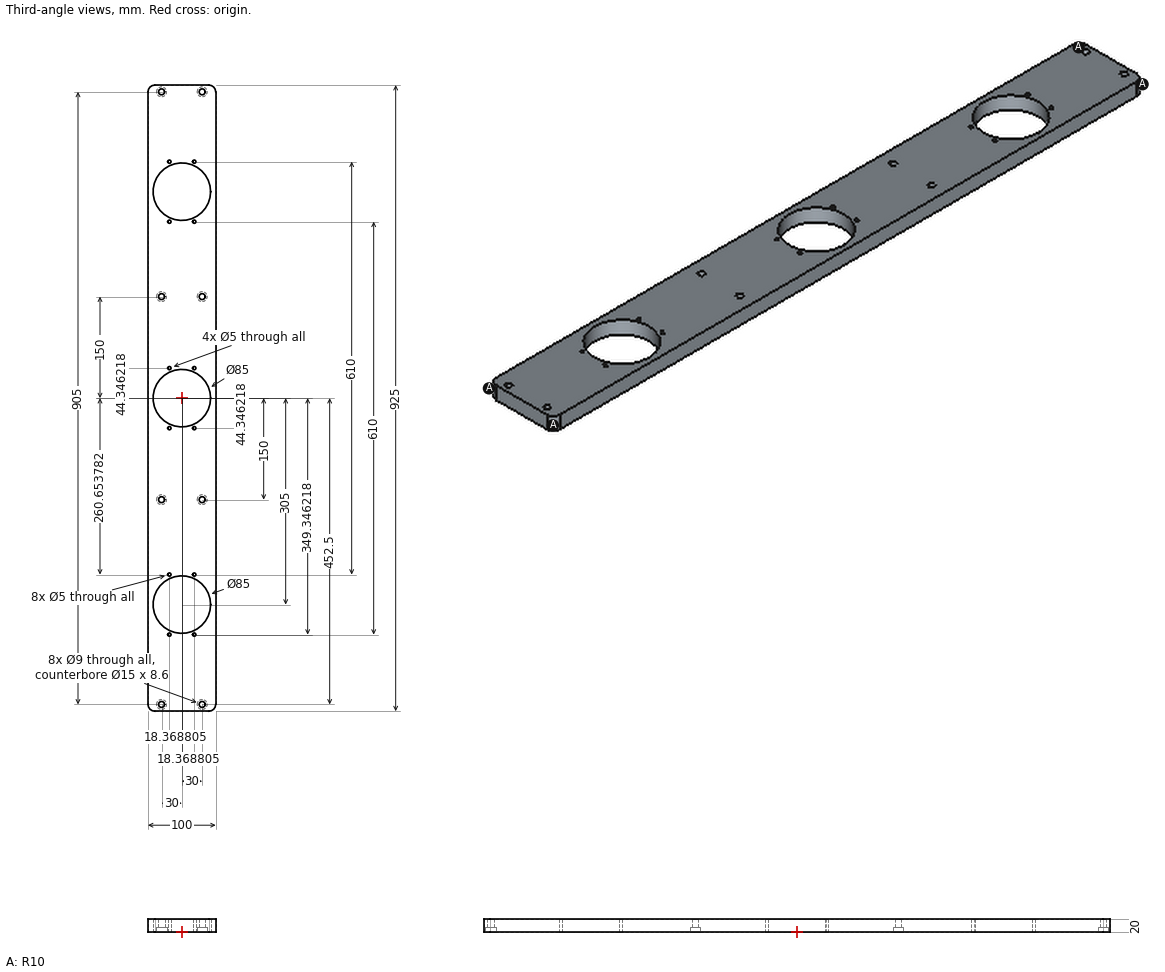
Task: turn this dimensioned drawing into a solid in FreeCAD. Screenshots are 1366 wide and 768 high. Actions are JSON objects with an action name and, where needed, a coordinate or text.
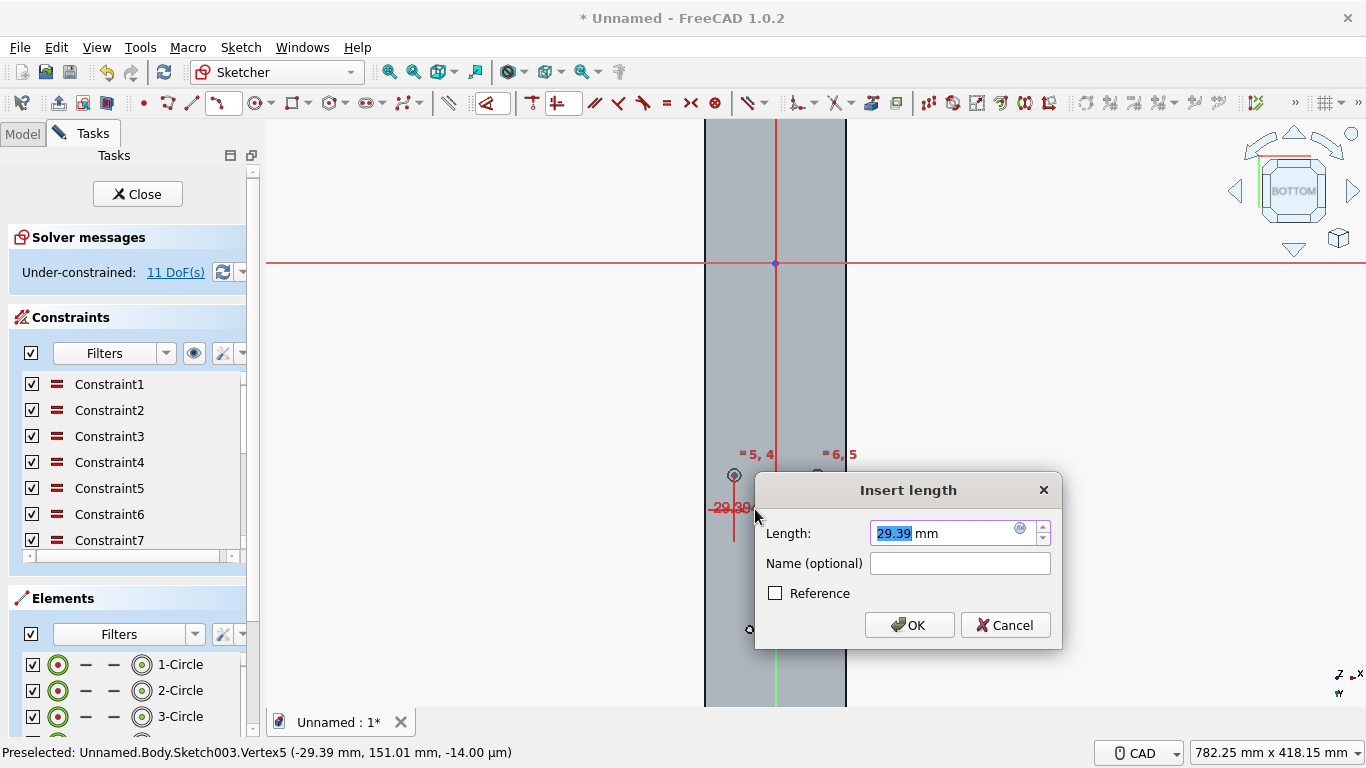
{"action": "type", "text": "30"}
{"action": "key", "text": "Return"}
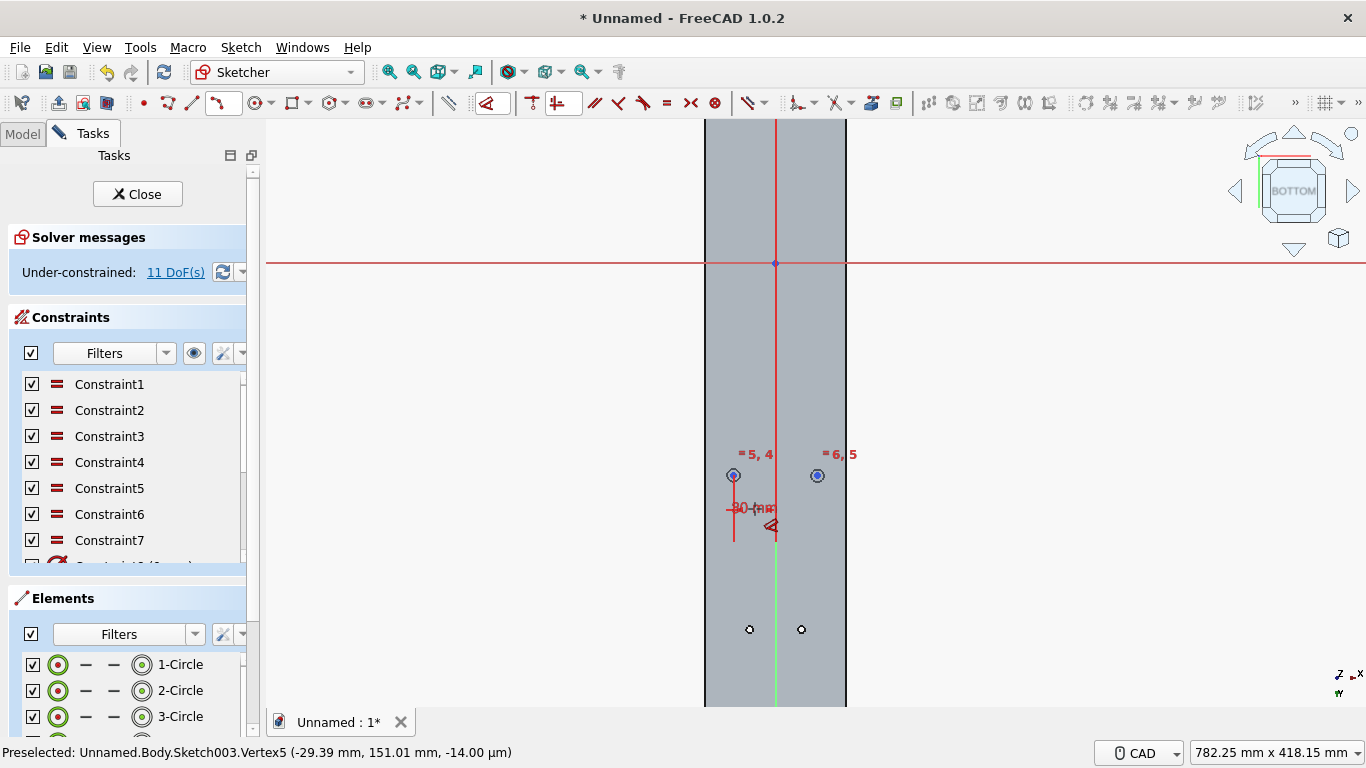
{"action": "left_click", "coordinate": [818, 476]}
{"action": "left_click", "coordinate": [797, 229]}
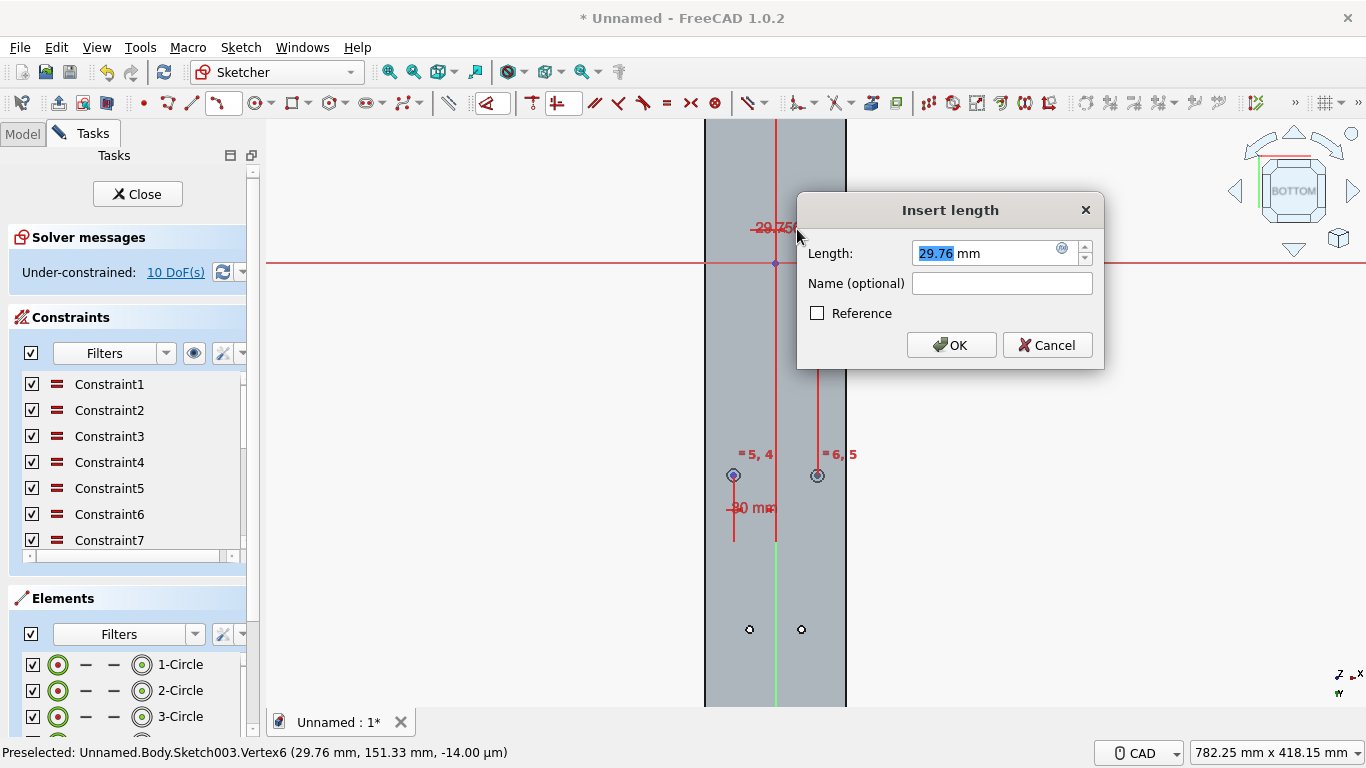
{"action": "type", "text": "30"}
{"action": "key", "text": "Return"}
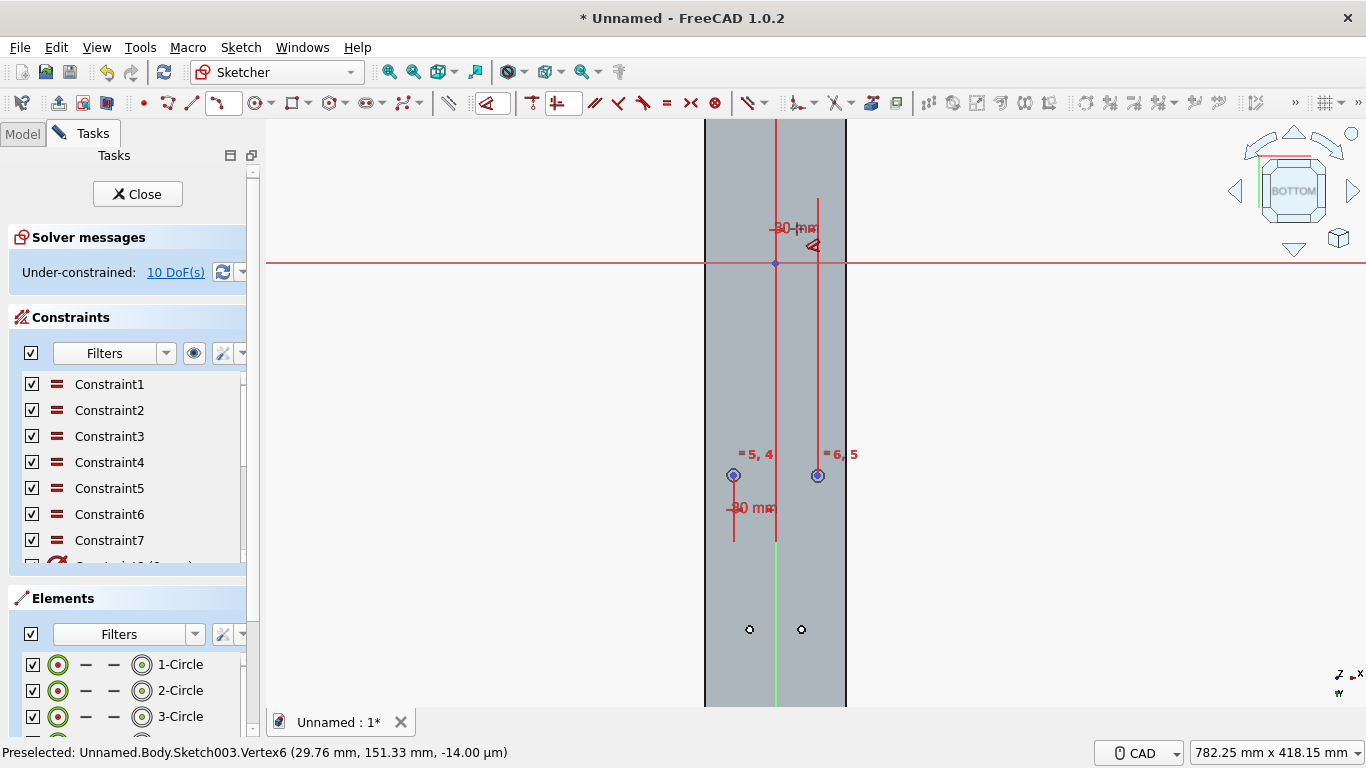
{"action": "scroll", "coordinate": [735, 478], "scroll_direction": "down", "scroll_amount": 6}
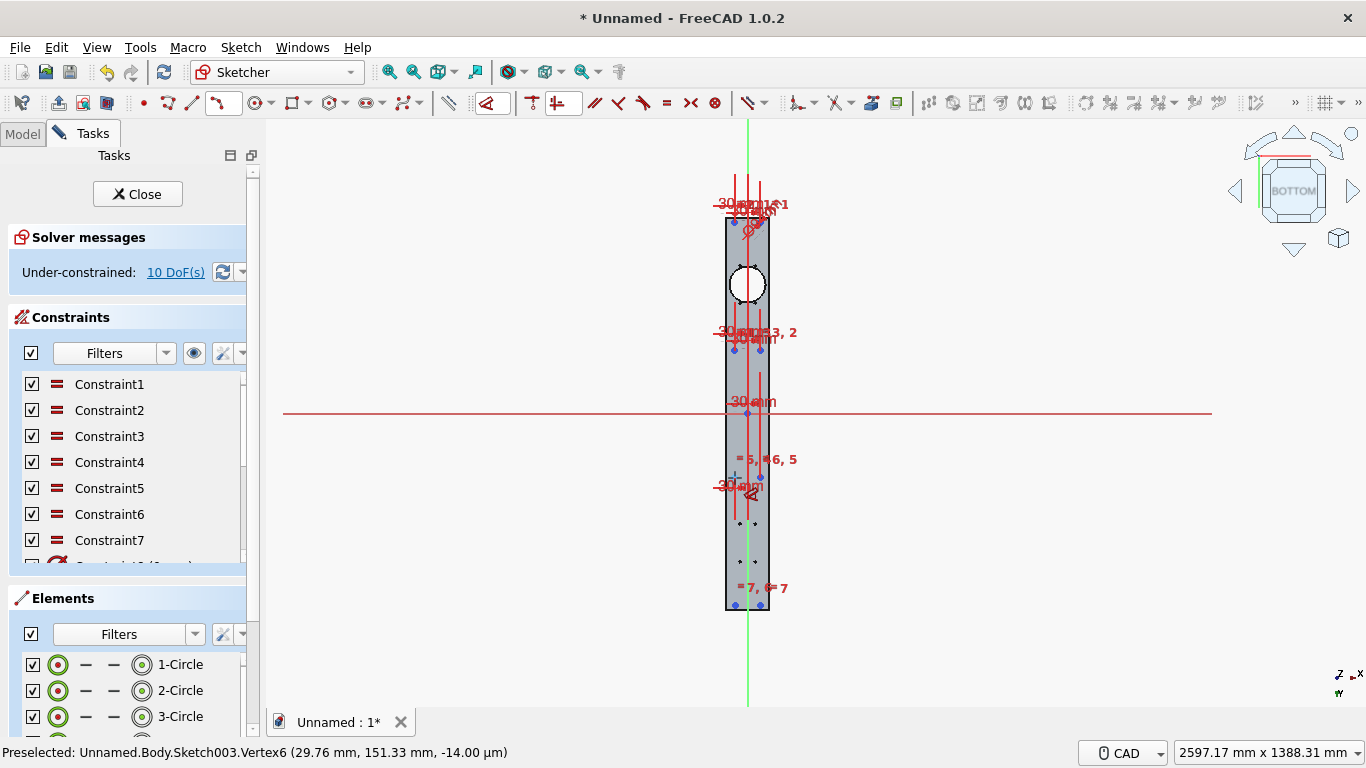
{"action": "scroll", "coordinate": [735, 606], "scroll_direction": "up", "scroll_amount": 6}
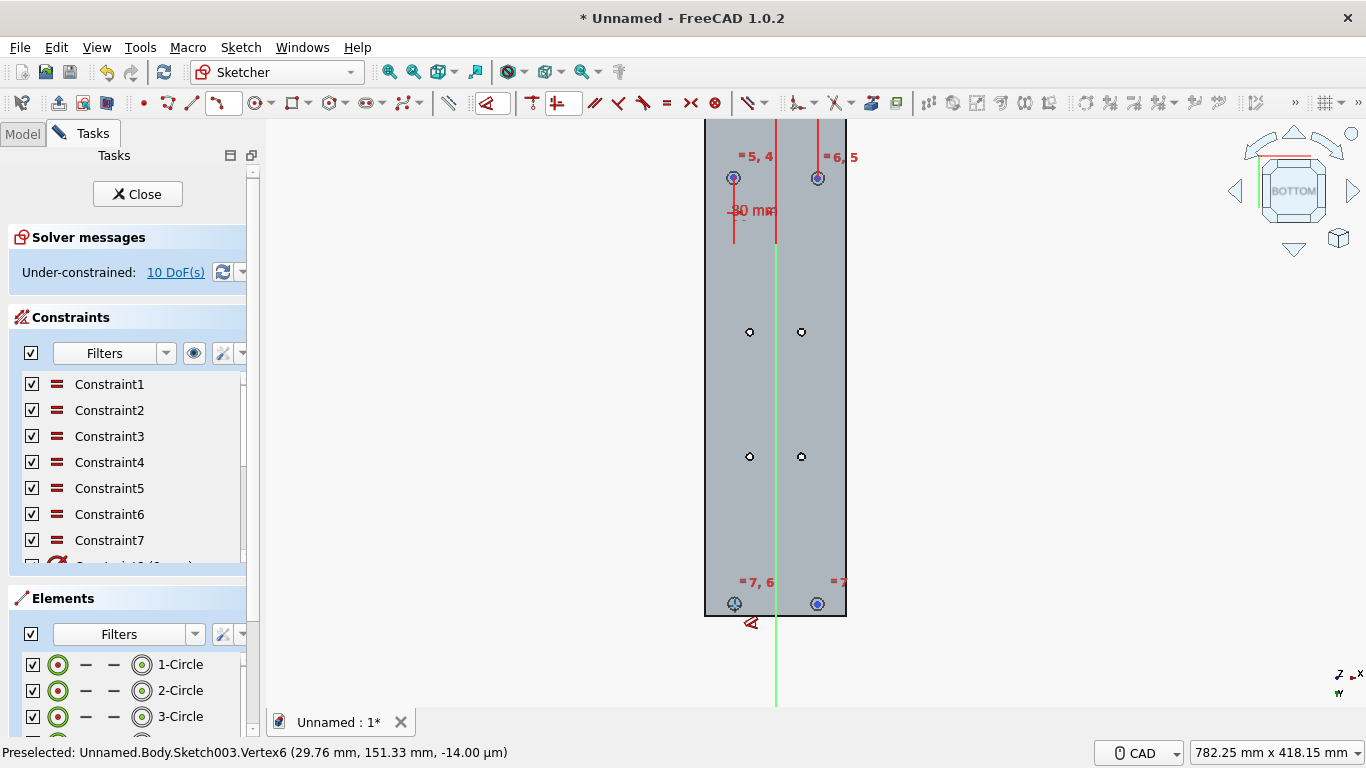
{"action": "left_click", "coordinate": [735, 604]}
{"action": "left_click", "coordinate": [755, 638]}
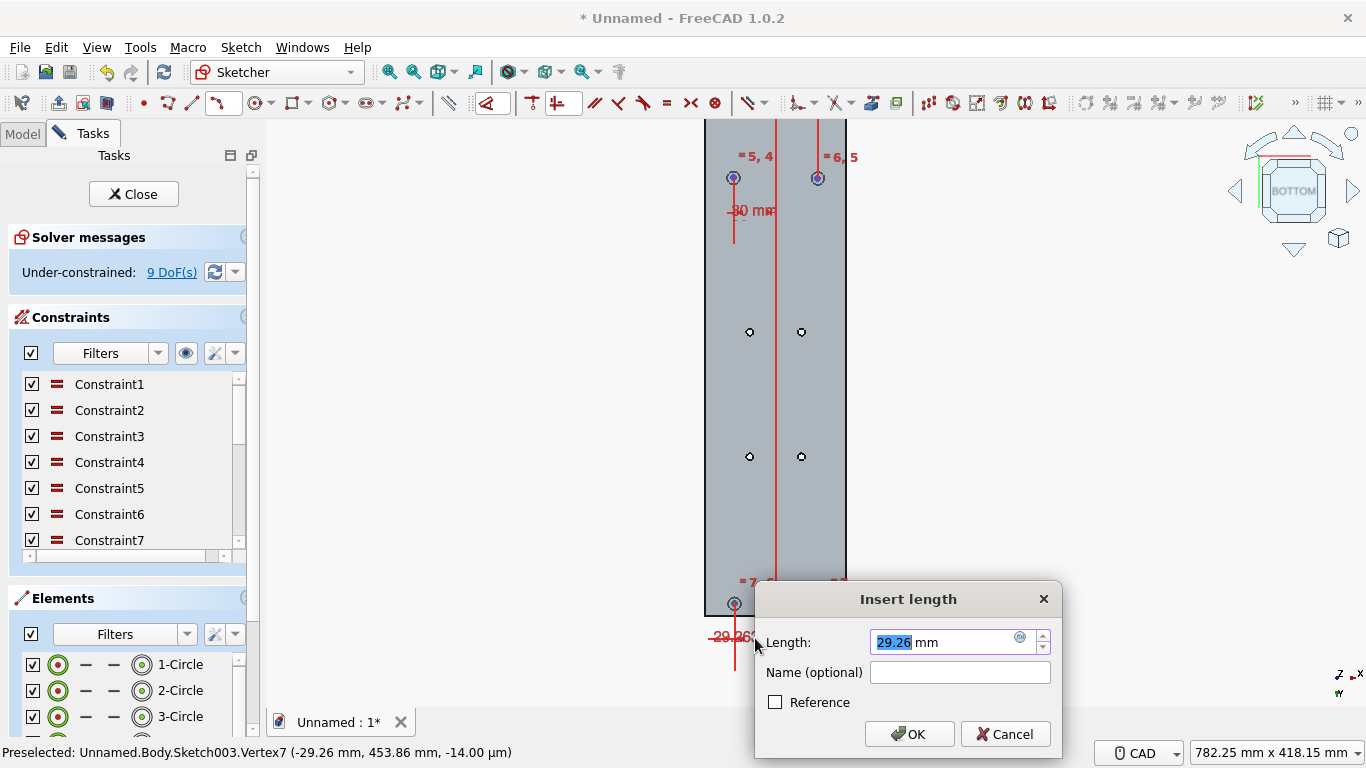
{"action": "type", "text": "30"}
{"action": "key", "text": "Return"}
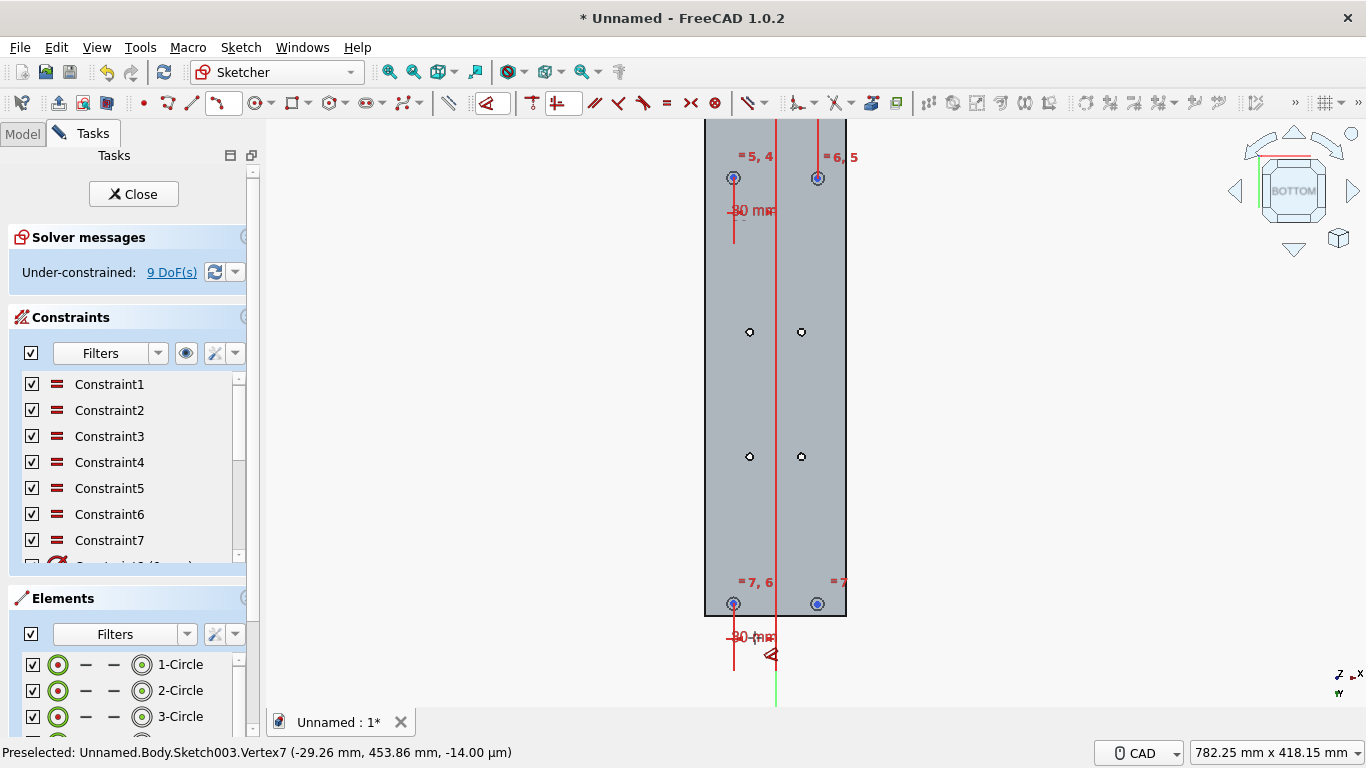
{"action": "left_click", "coordinate": [817, 604]}
{"action": "left_click", "coordinate": [797, 662]}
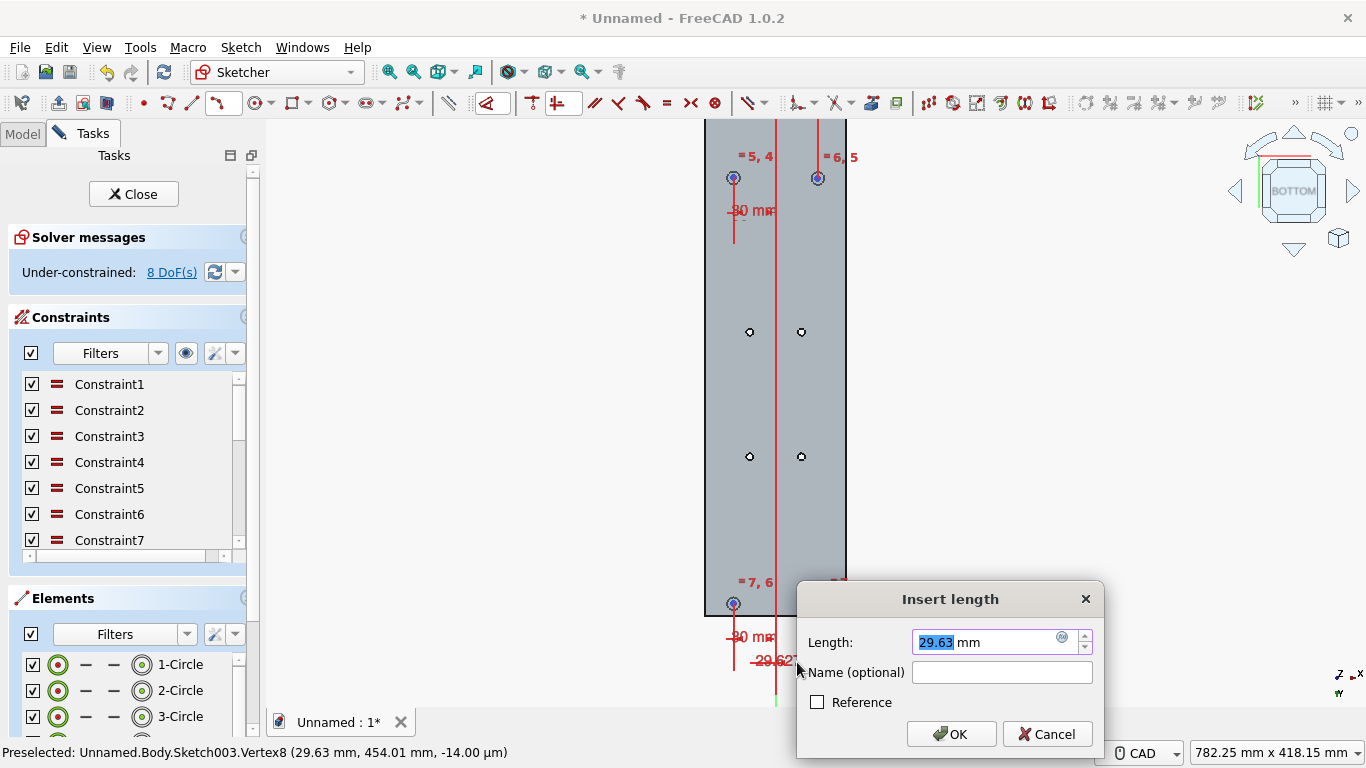
{"action": "type", "text": "30"}
{"action": "key", "text": "Return"}